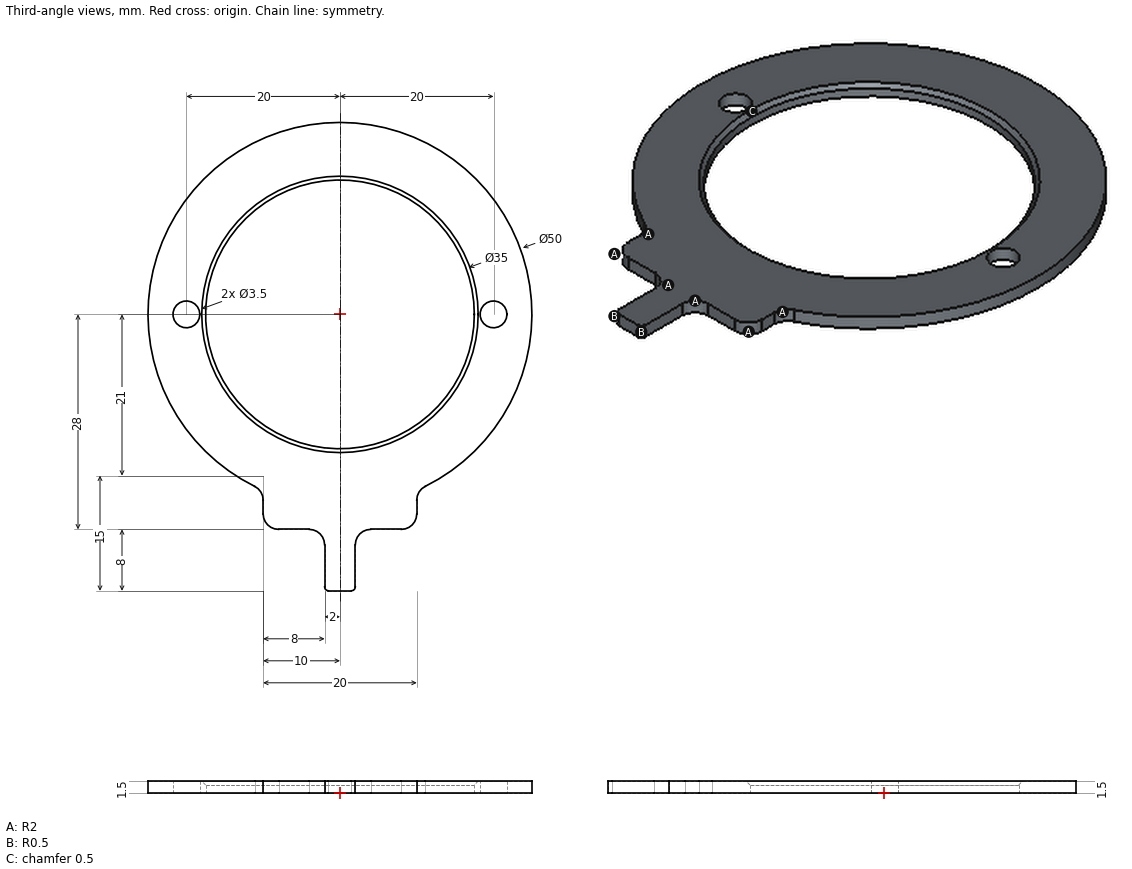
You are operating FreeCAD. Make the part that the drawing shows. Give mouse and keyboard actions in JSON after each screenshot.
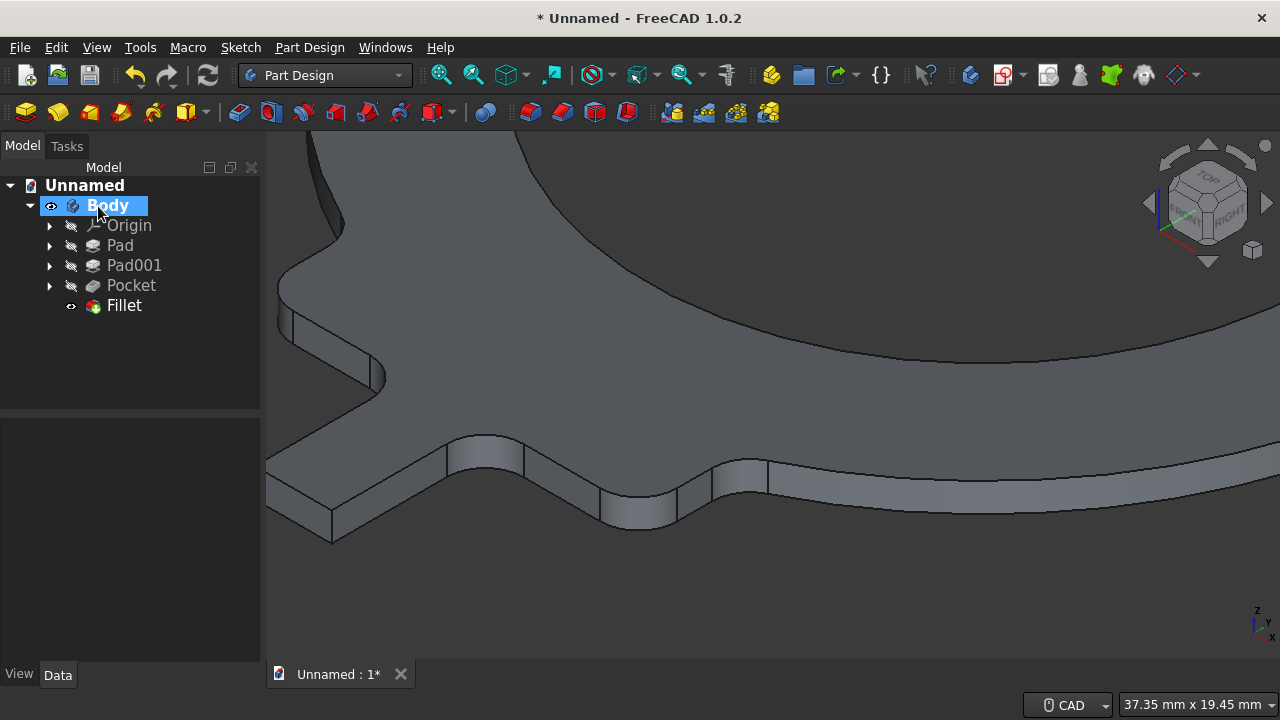
{"action": "left_click", "coordinate": [442, 76]}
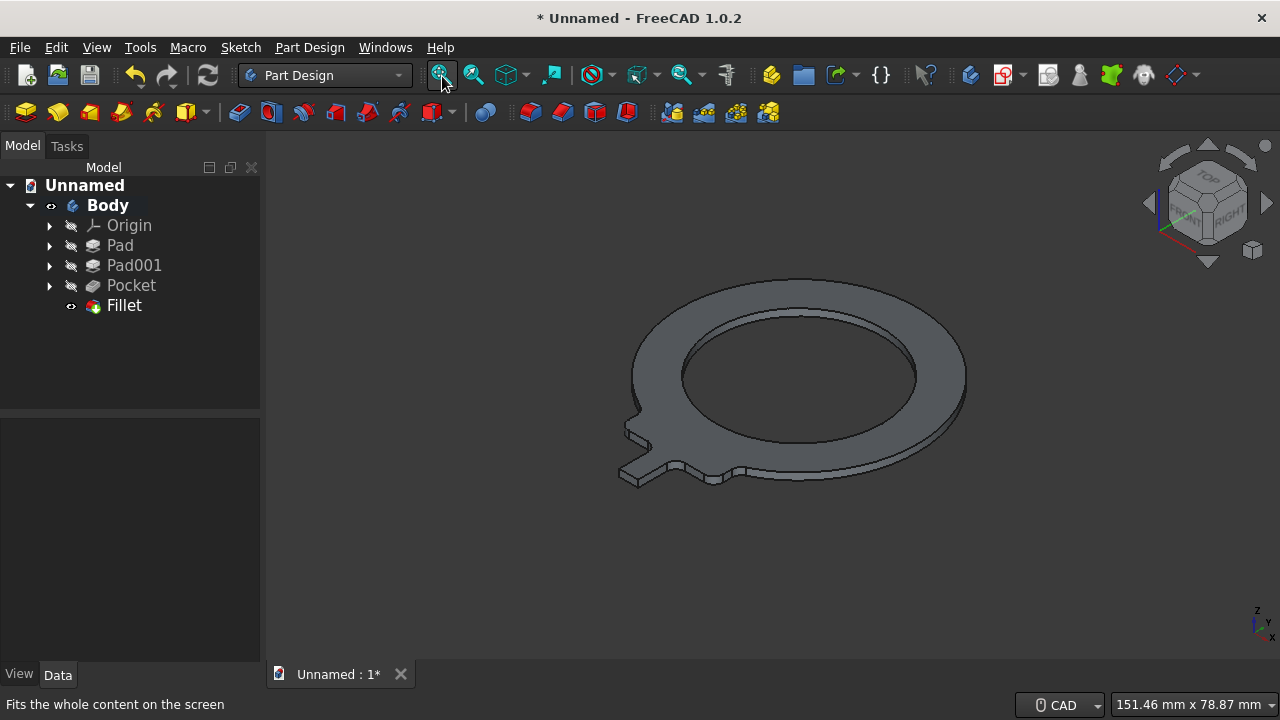
{"action": "left_click", "coordinate": [691, 437]}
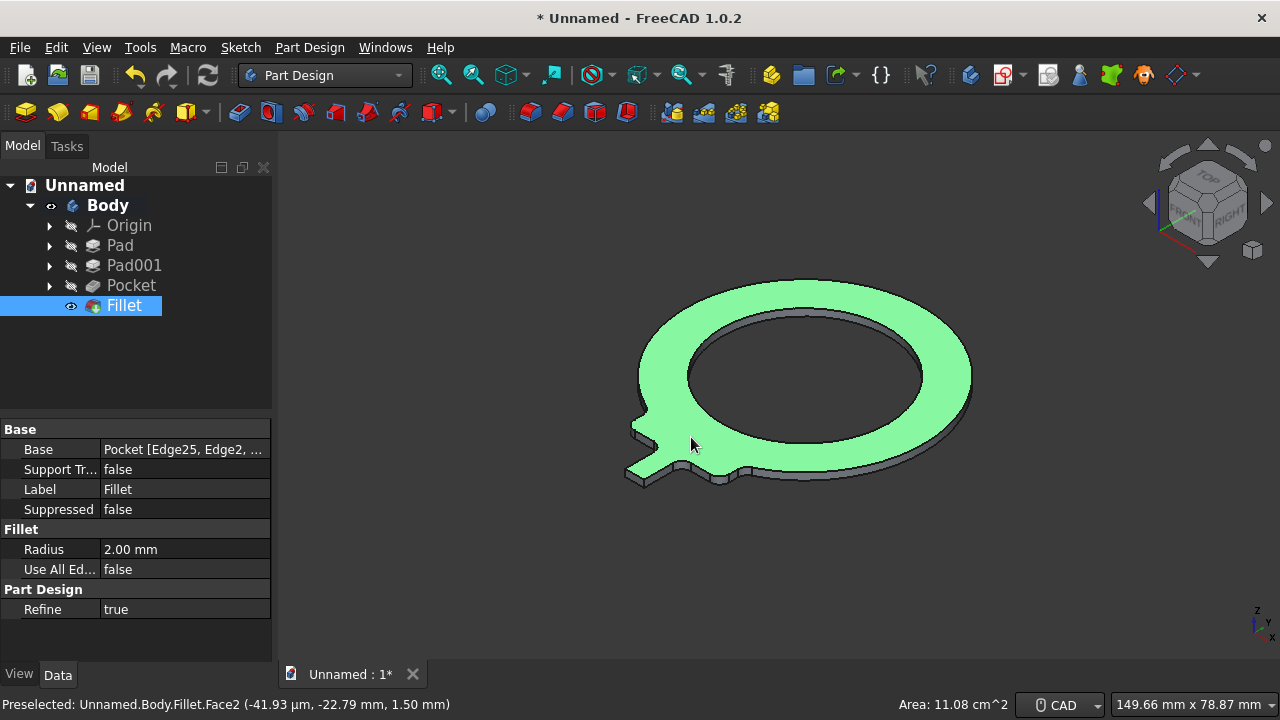
{"action": "left_click", "coordinate": [1004, 76]}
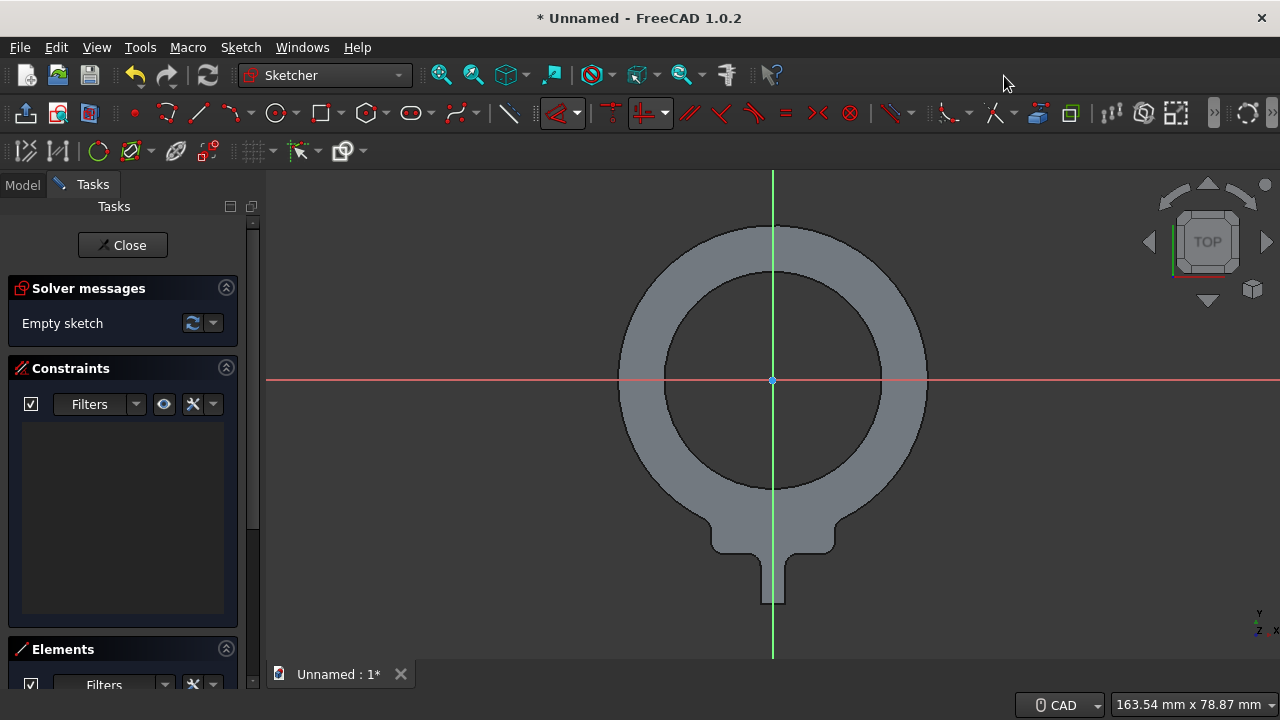
{"action": "scroll", "coordinate": [829, 352], "scroll_direction": "up", "scroll_amount": 4}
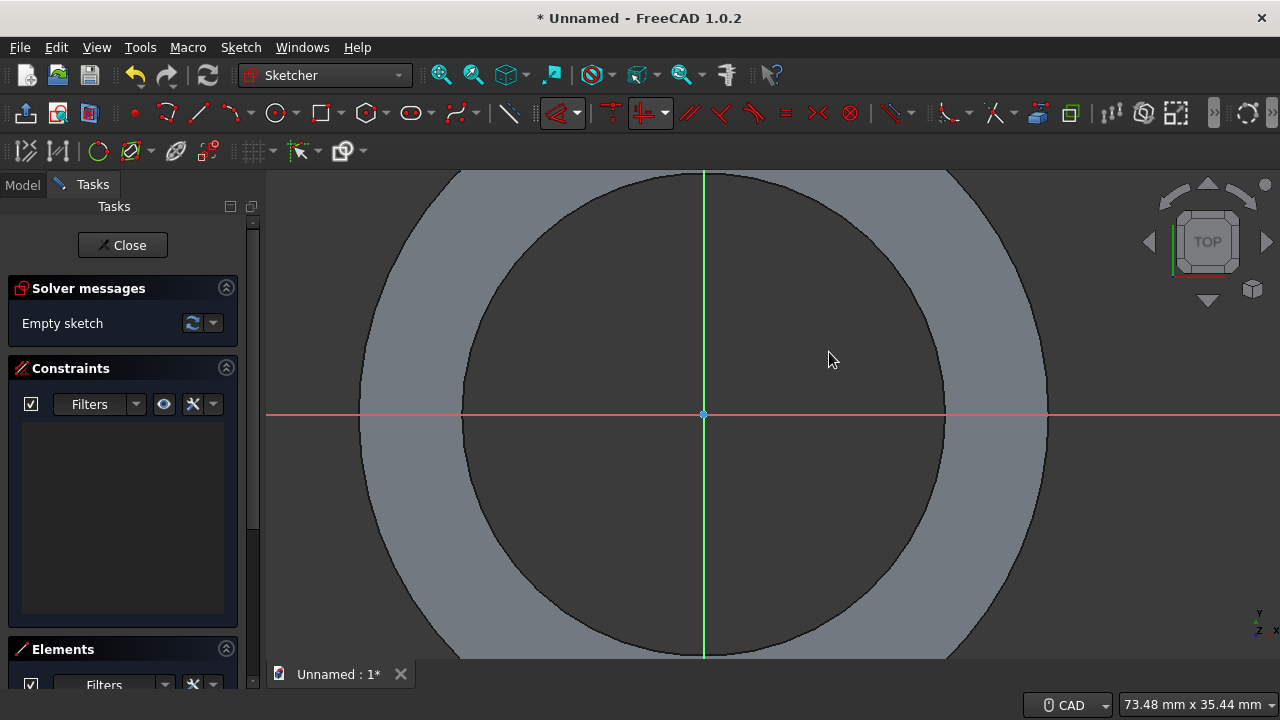
{"action": "left_click", "coordinate": [276, 114]}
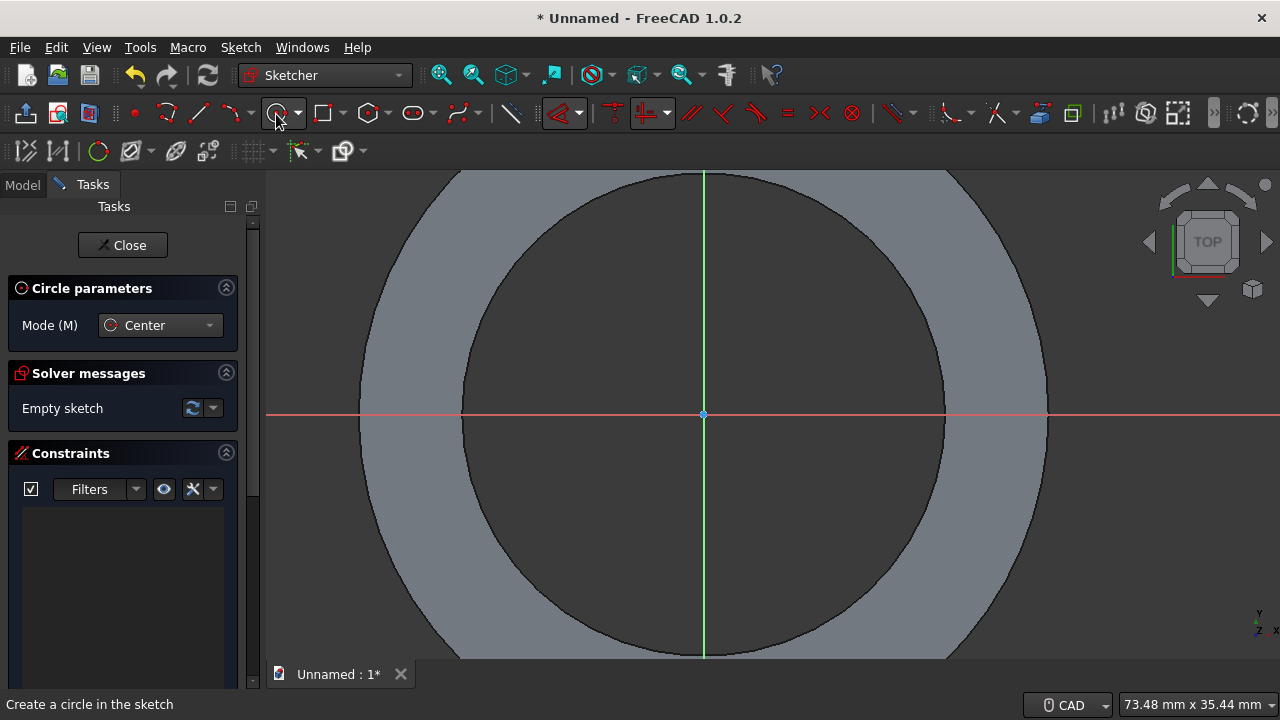
{"action": "left_click", "coordinate": [428, 415]}
{"action": "left_click", "coordinate": [445, 397]}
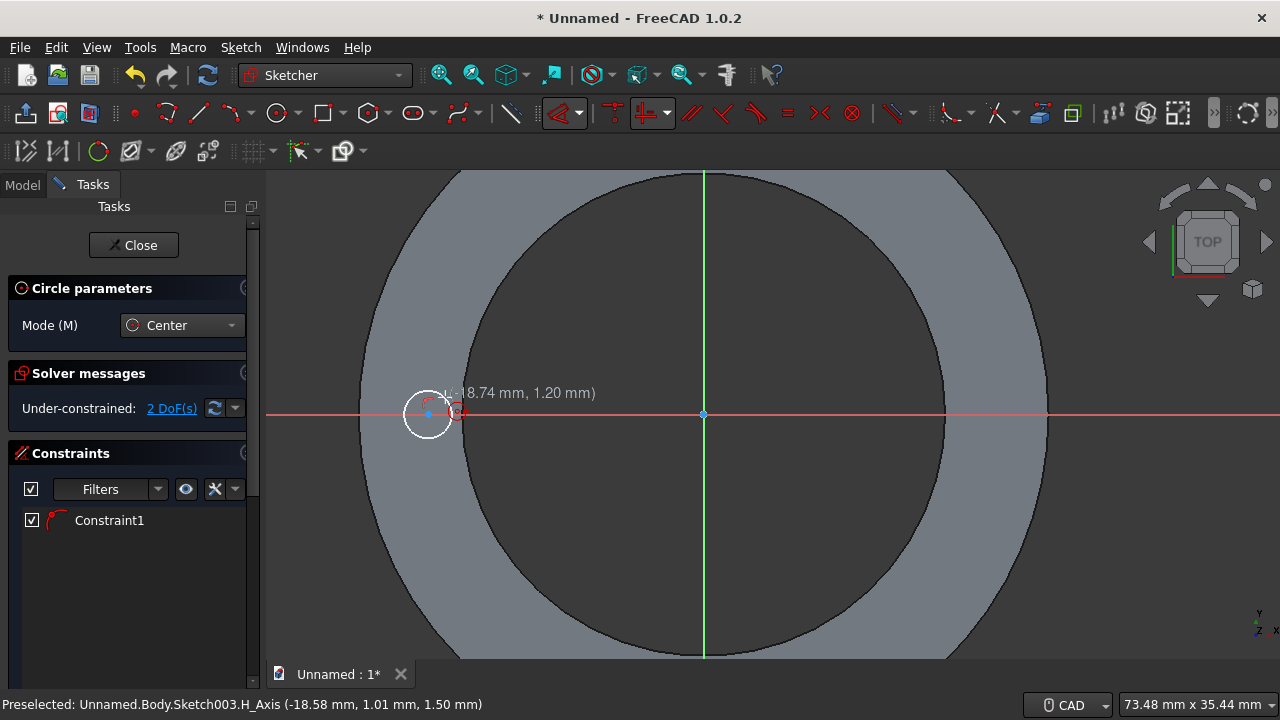
{"action": "left_click", "coordinate": [980, 415]}
{"action": "left_click", "coordinate": [997, 397]}
{"action": "key", "text": "Escape"}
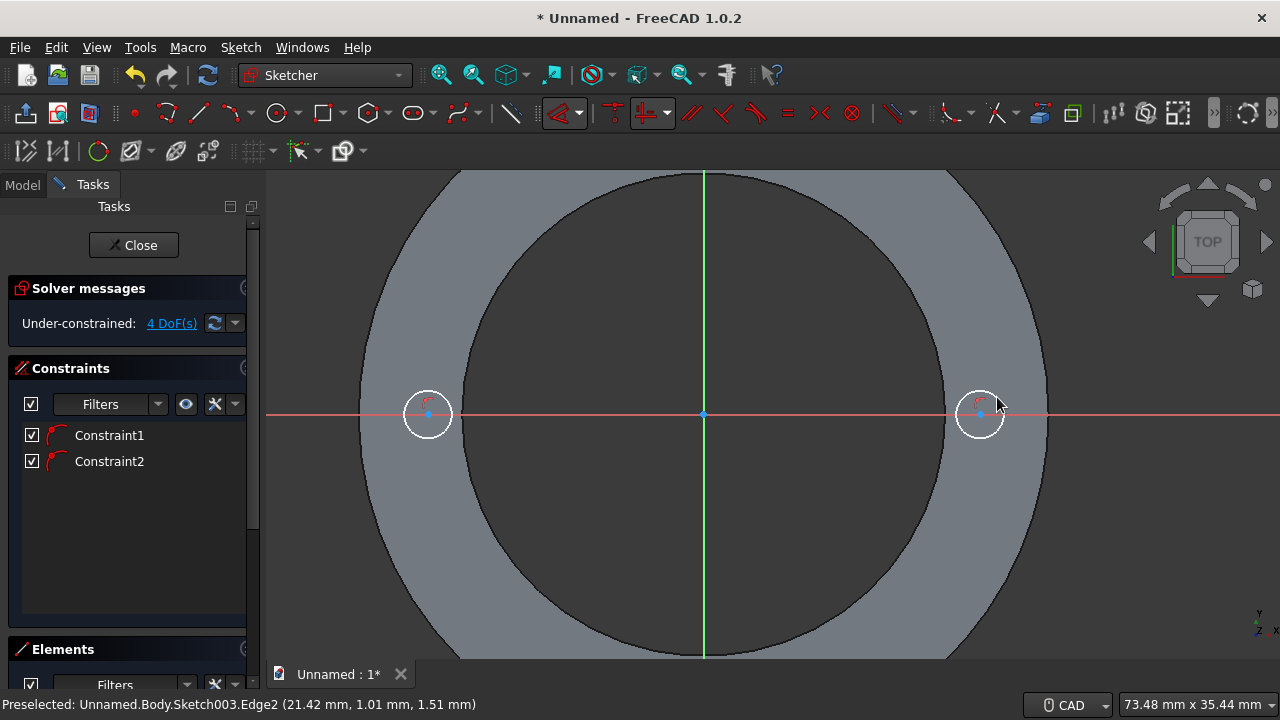
{"action": "left_click", "coordinate": [445, 398]}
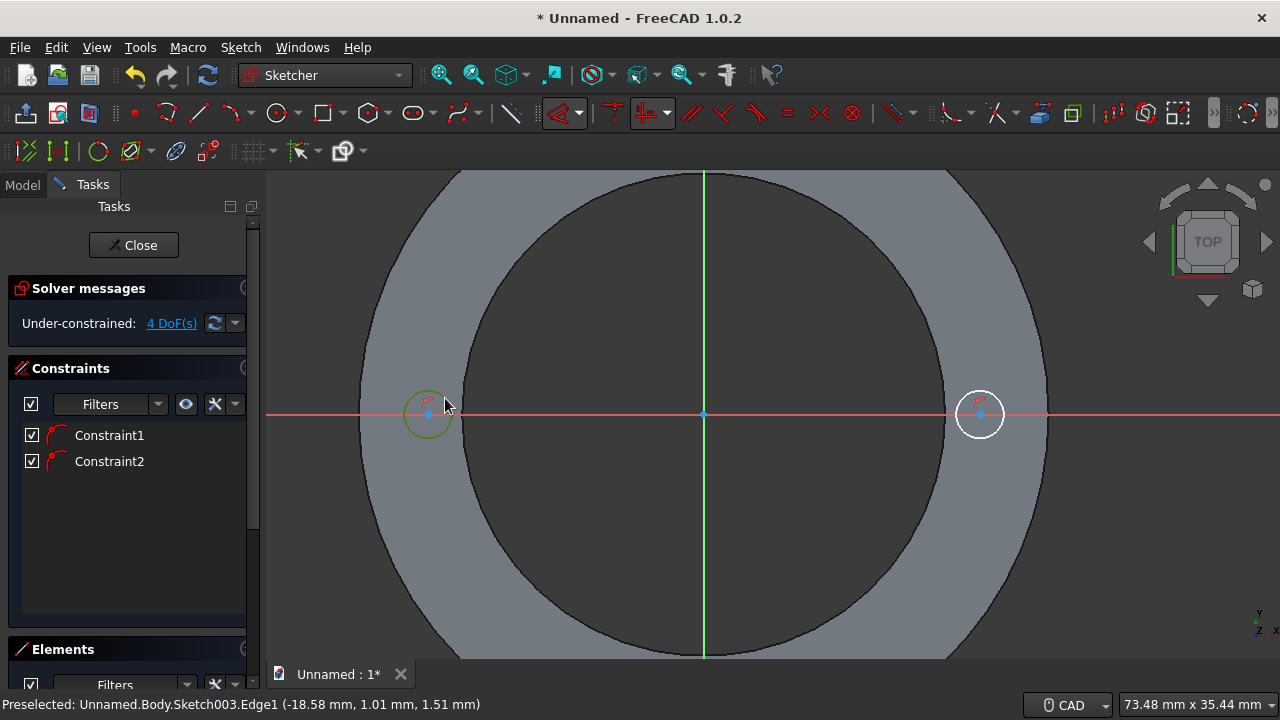
{"action": "left_click", "coordinate": [997, 398]}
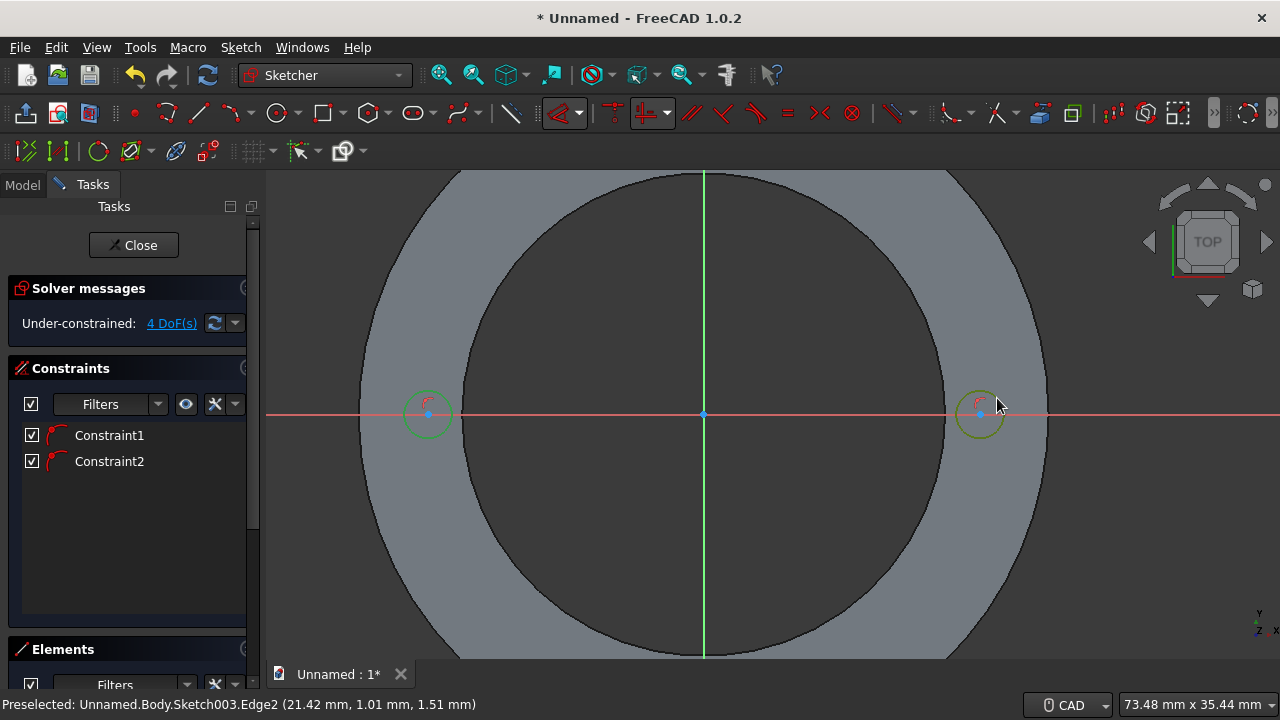
{"action": "left_click", "coordinate": [788, 114]}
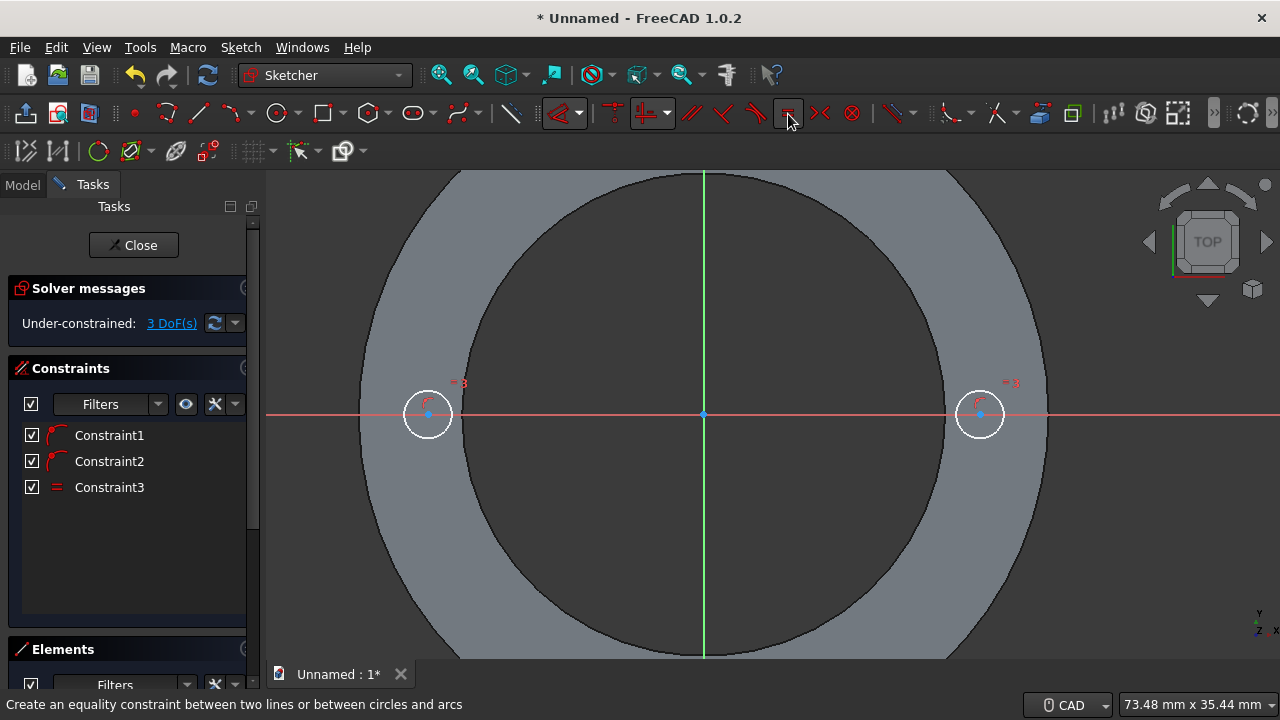
{"action": "left_click", "coordinate": [445, 398]}